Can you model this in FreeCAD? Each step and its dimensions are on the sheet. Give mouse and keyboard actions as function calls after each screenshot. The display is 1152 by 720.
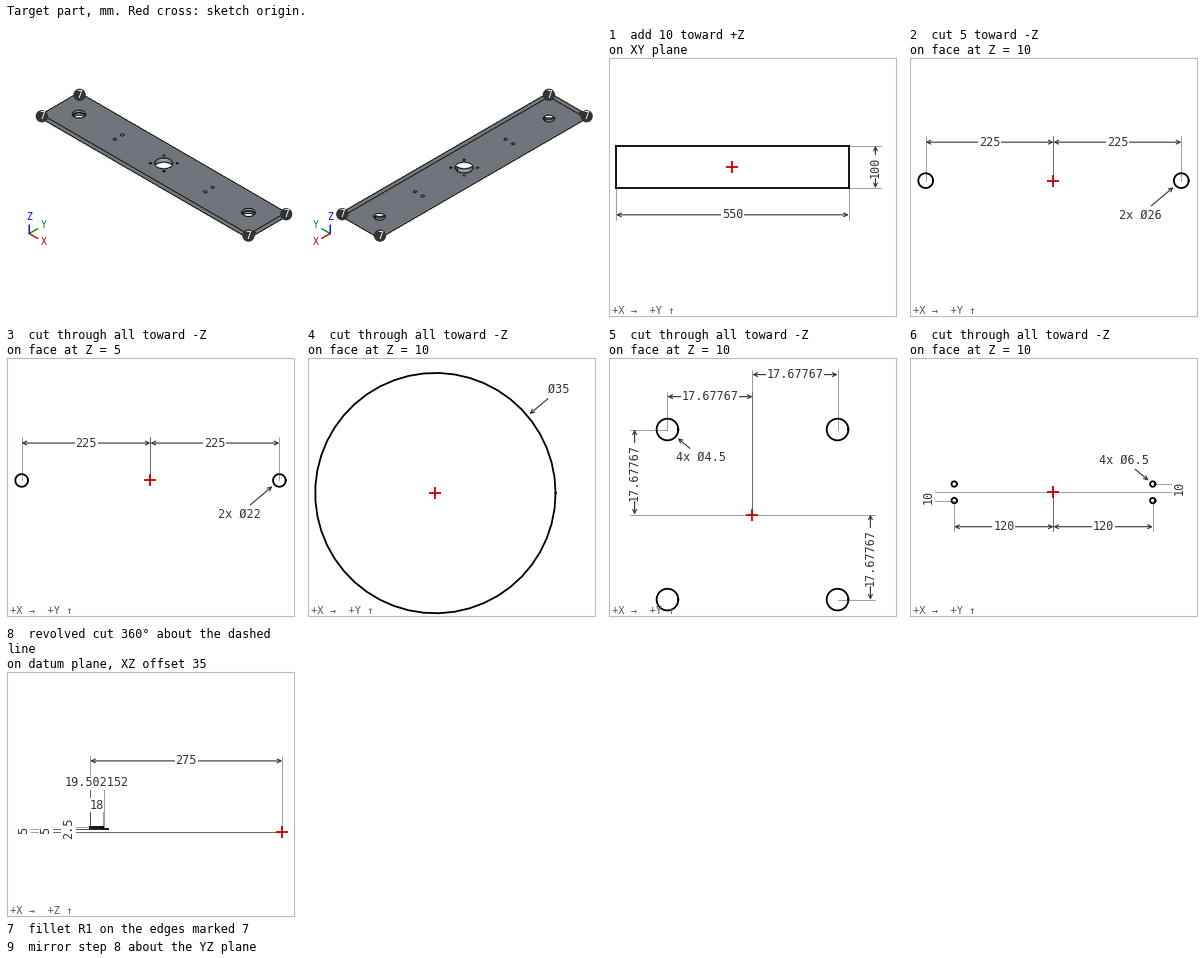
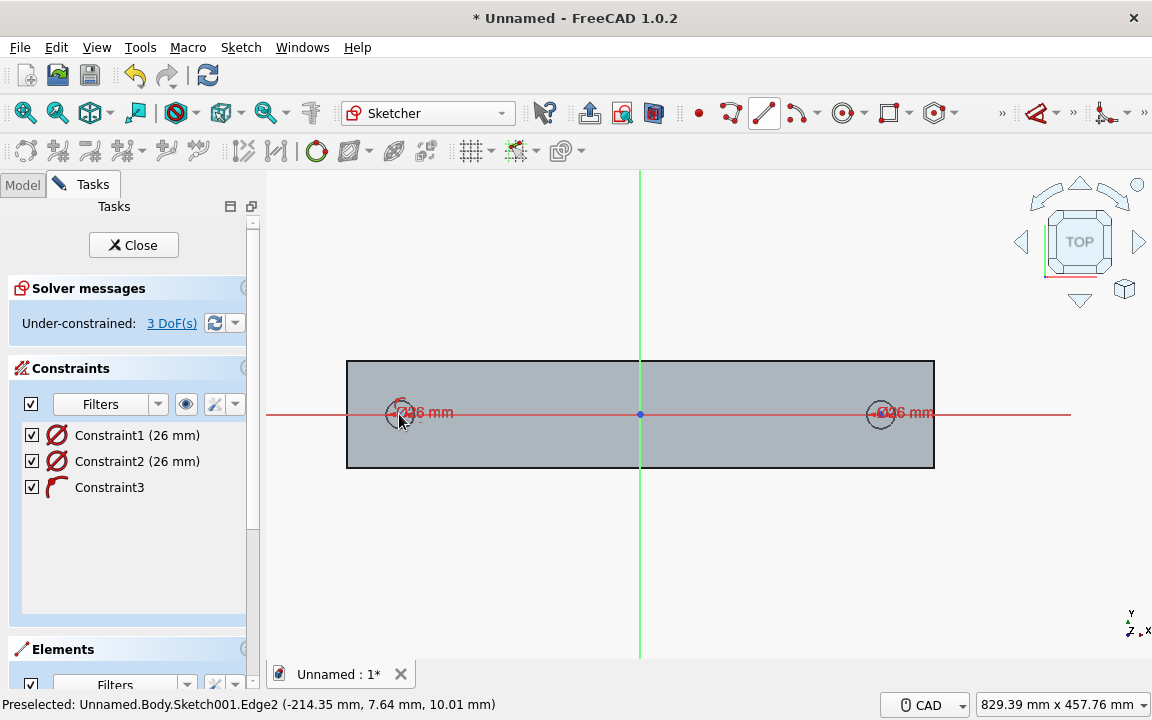
click(881, 415)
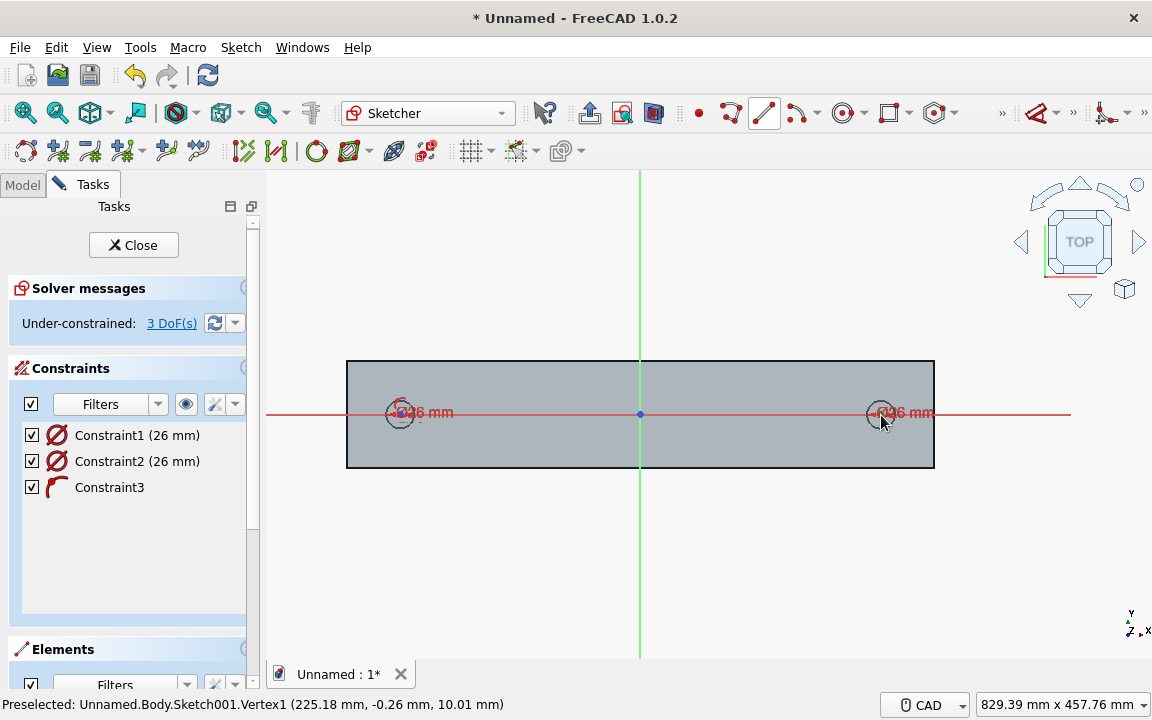
click(344, 414)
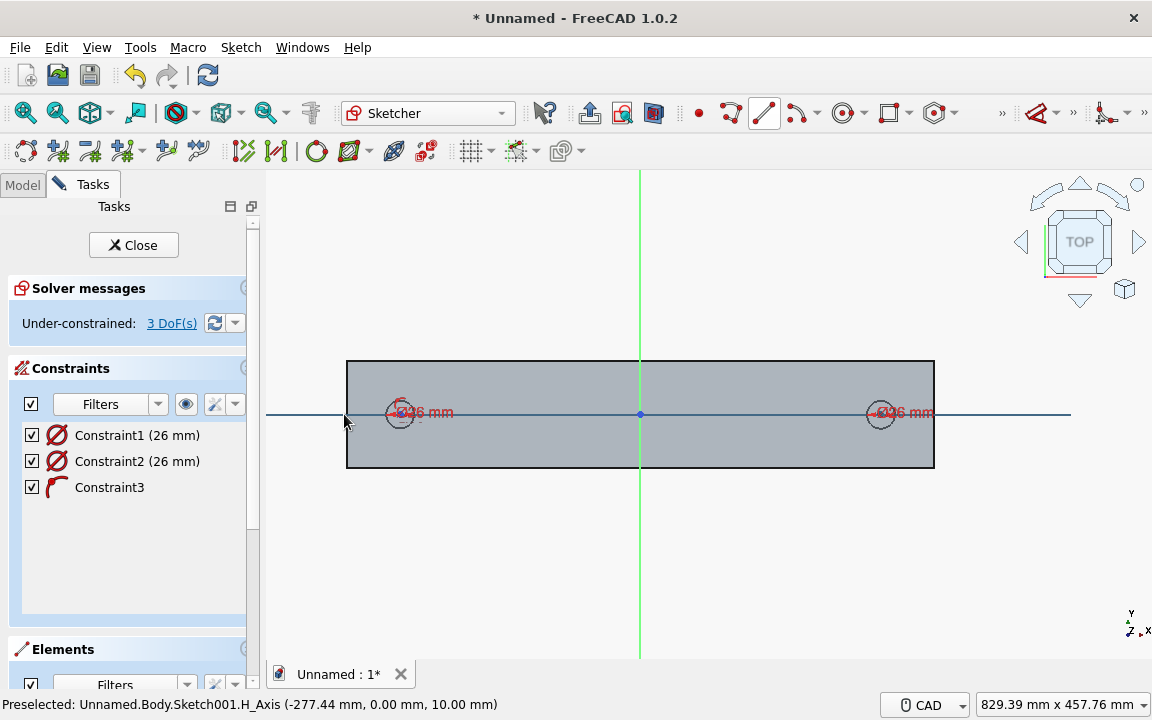
key(c)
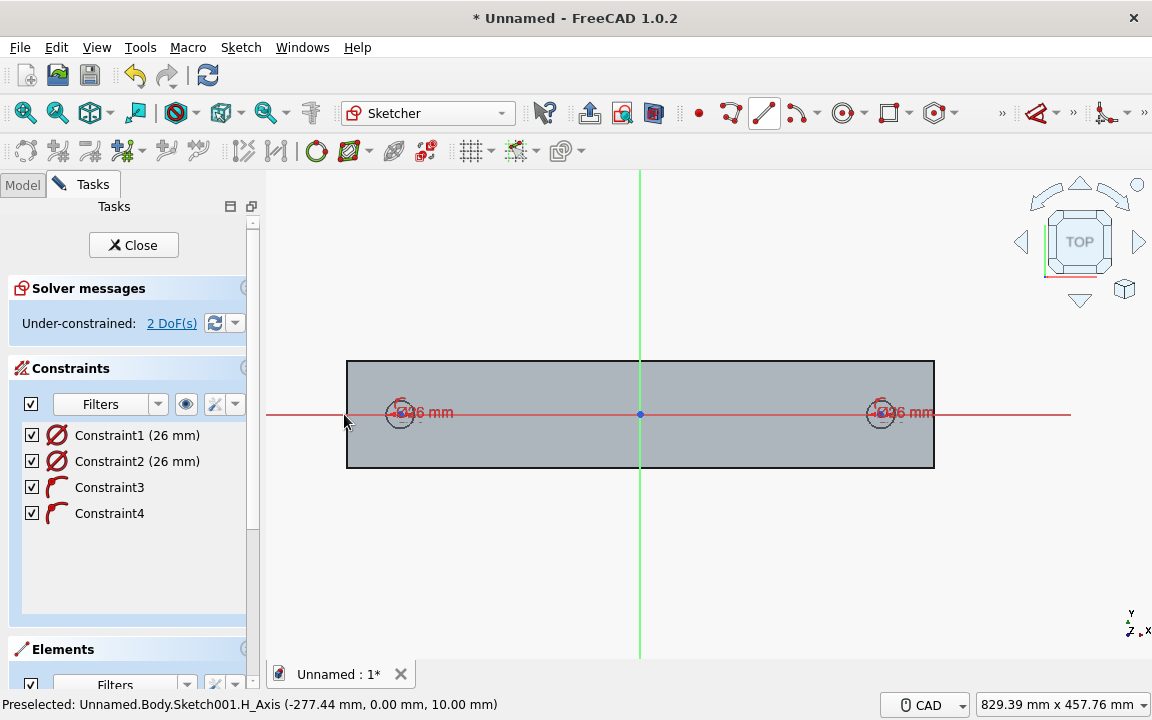
click(1036, 114)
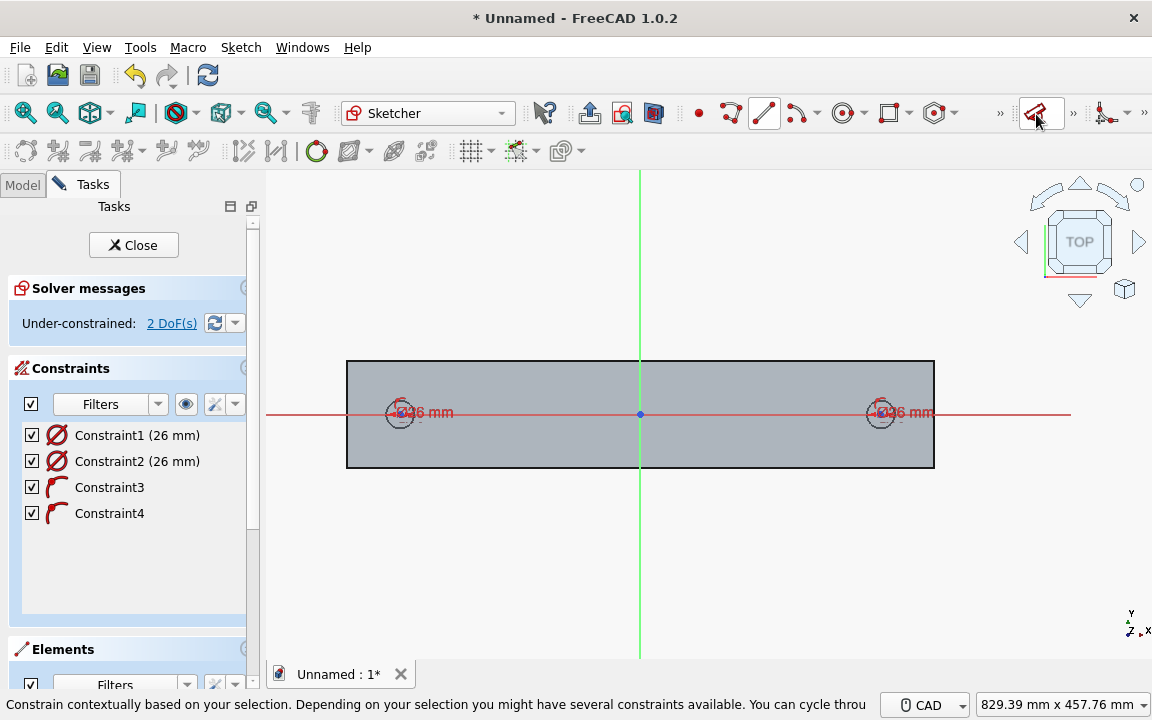
click(881, 414)
click(761, 448)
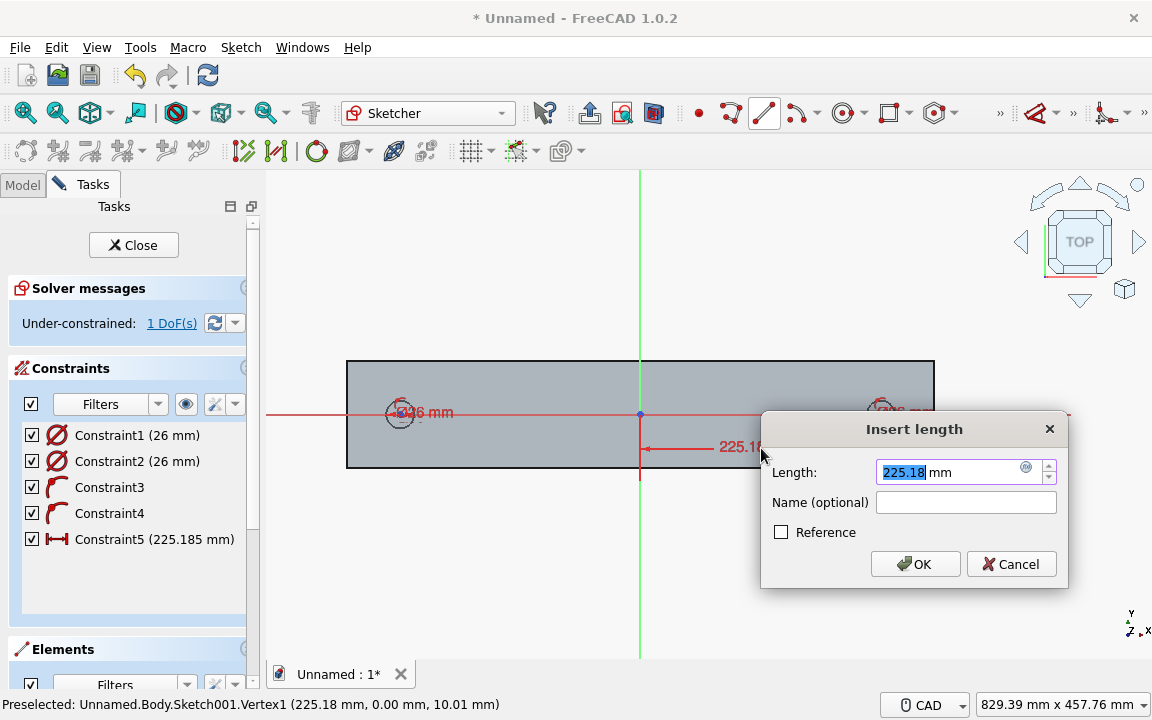
text(225)
key(Return)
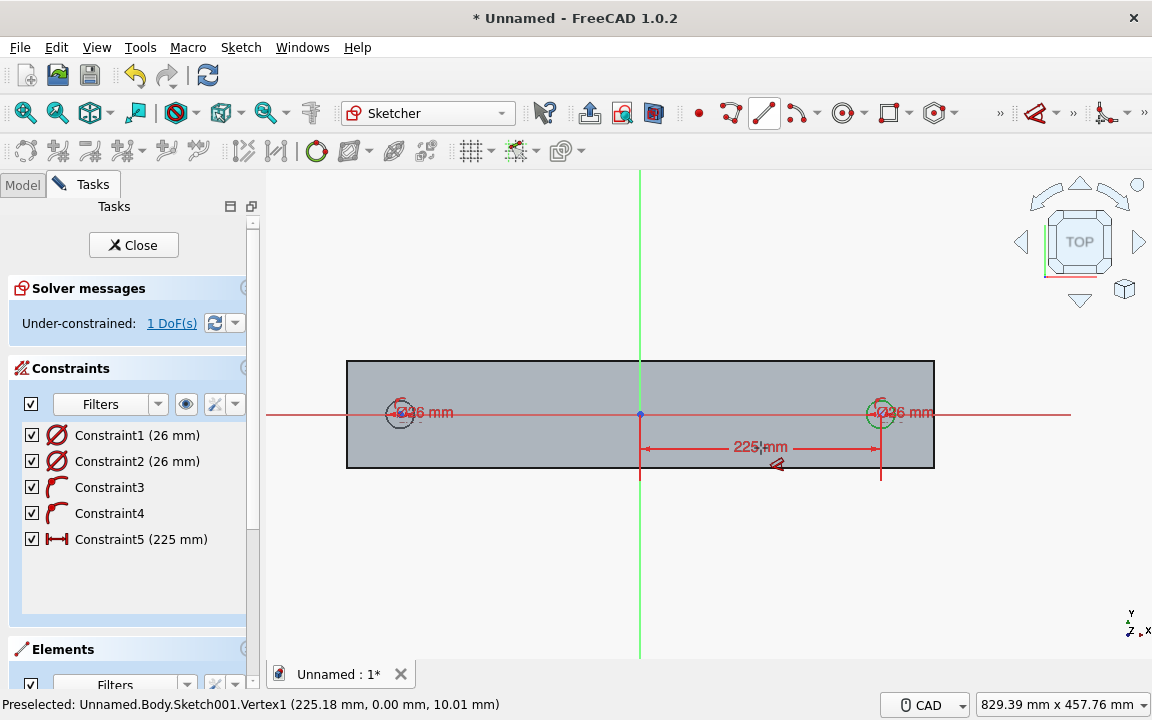
click(400, 414)
click(520, 448)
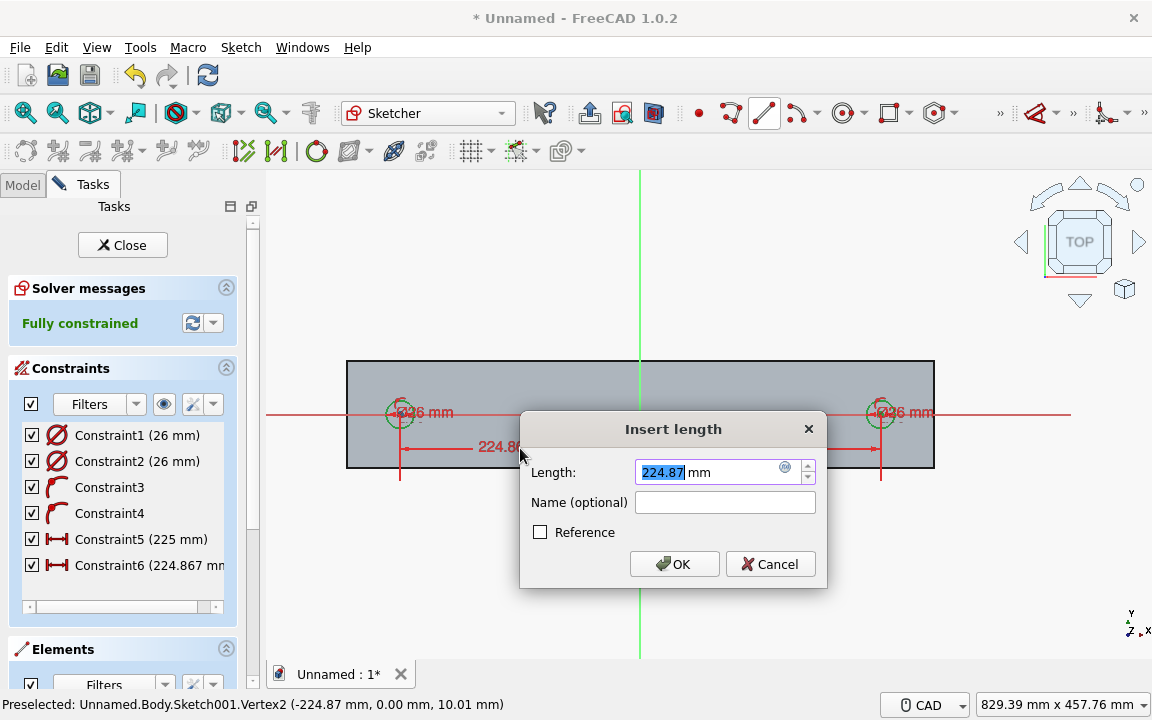
text(225)
key(Return)
key(Escape)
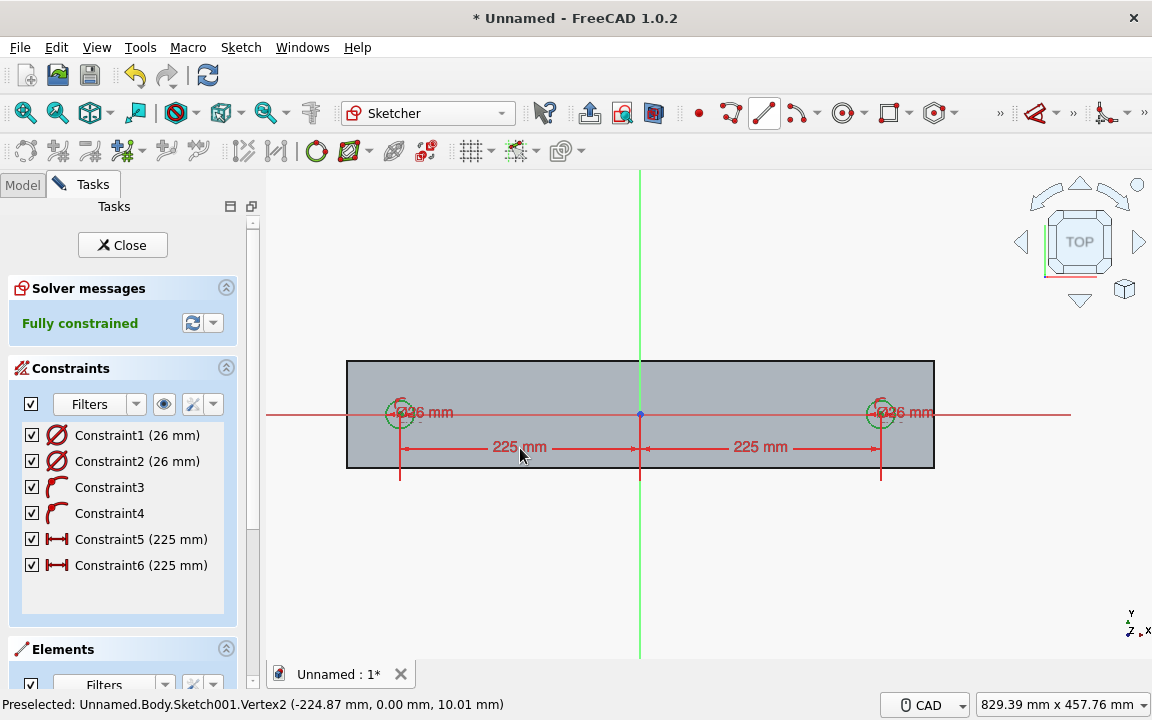
click(123, 245)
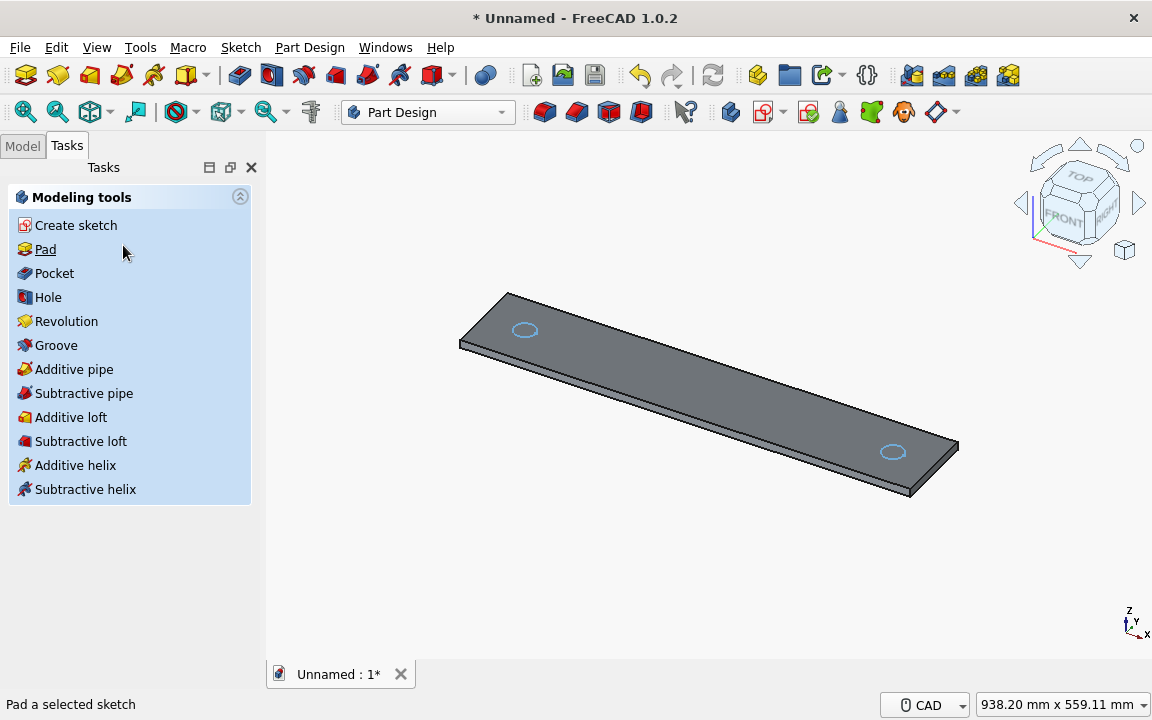
click(240, 76)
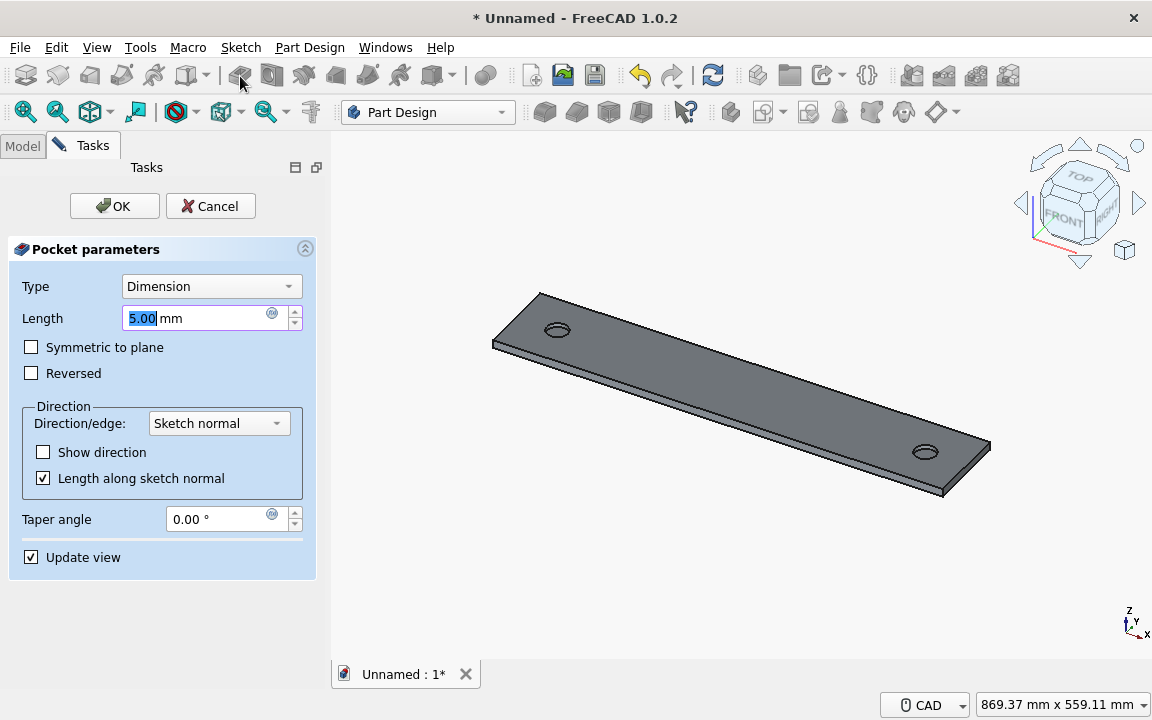
text(5)
key(Tab)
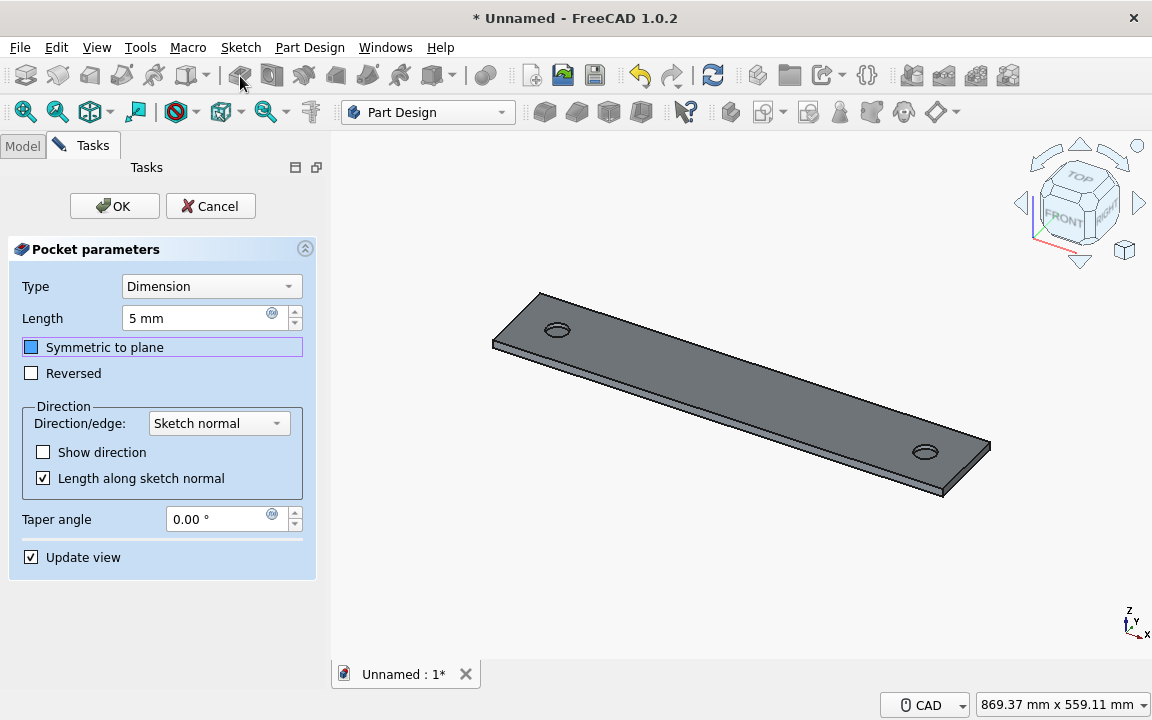
click(115, 206)